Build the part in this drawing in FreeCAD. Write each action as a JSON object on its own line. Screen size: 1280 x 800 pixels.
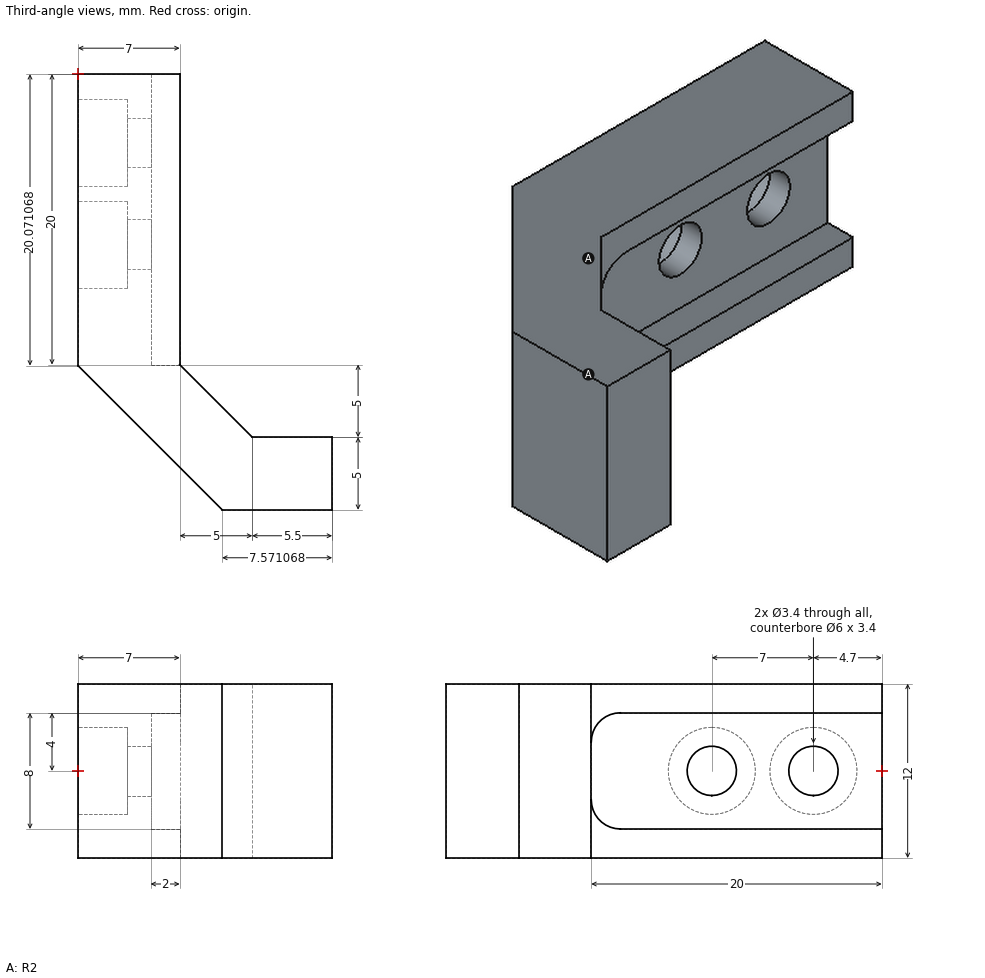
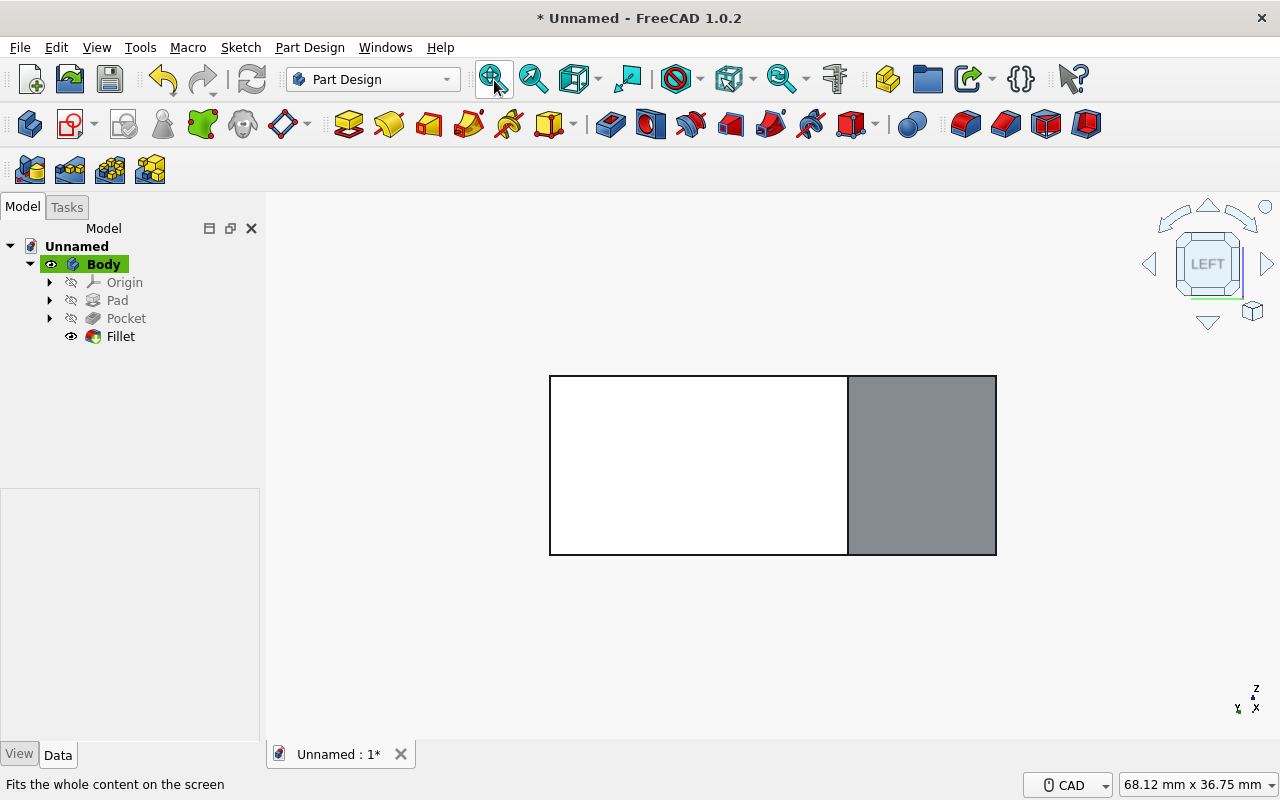
{"action": "left_click", "coordinate": [656, 464]}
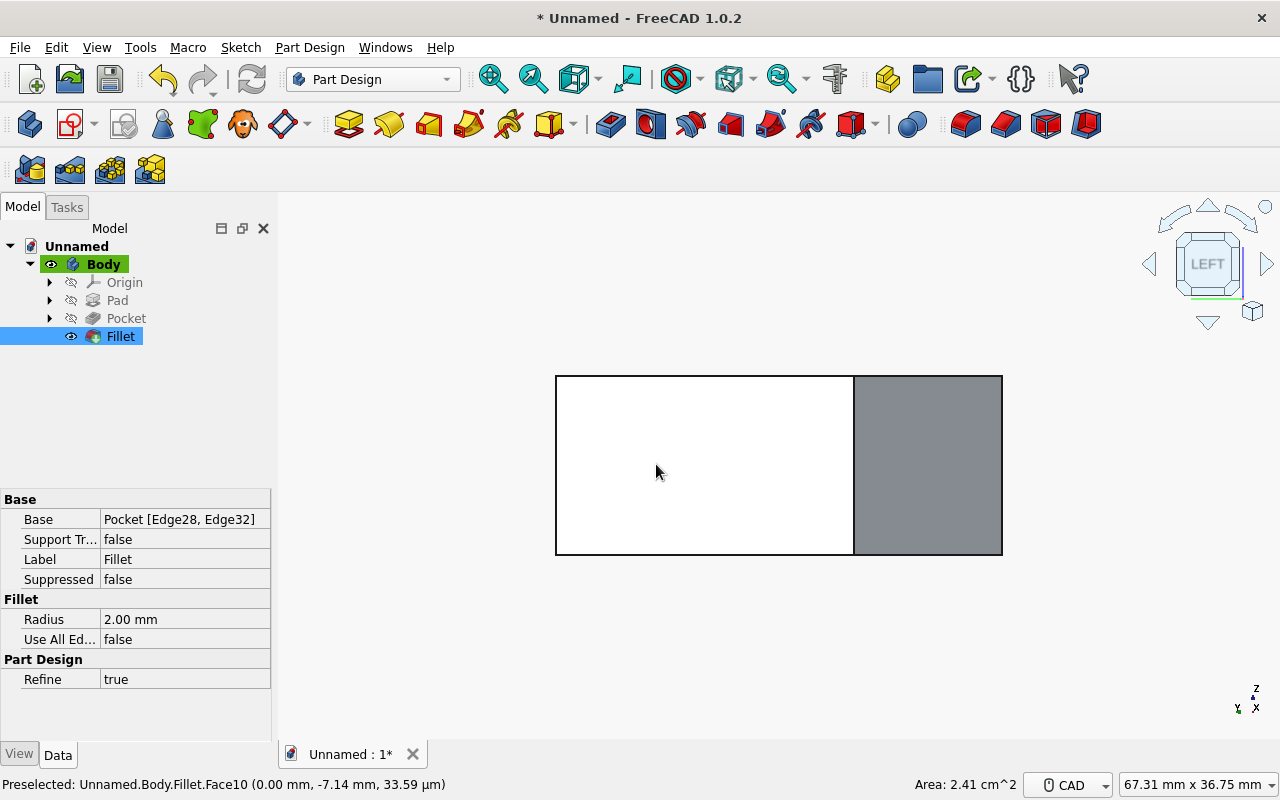
{"action": "left_click", "coordinate": [70, 124]}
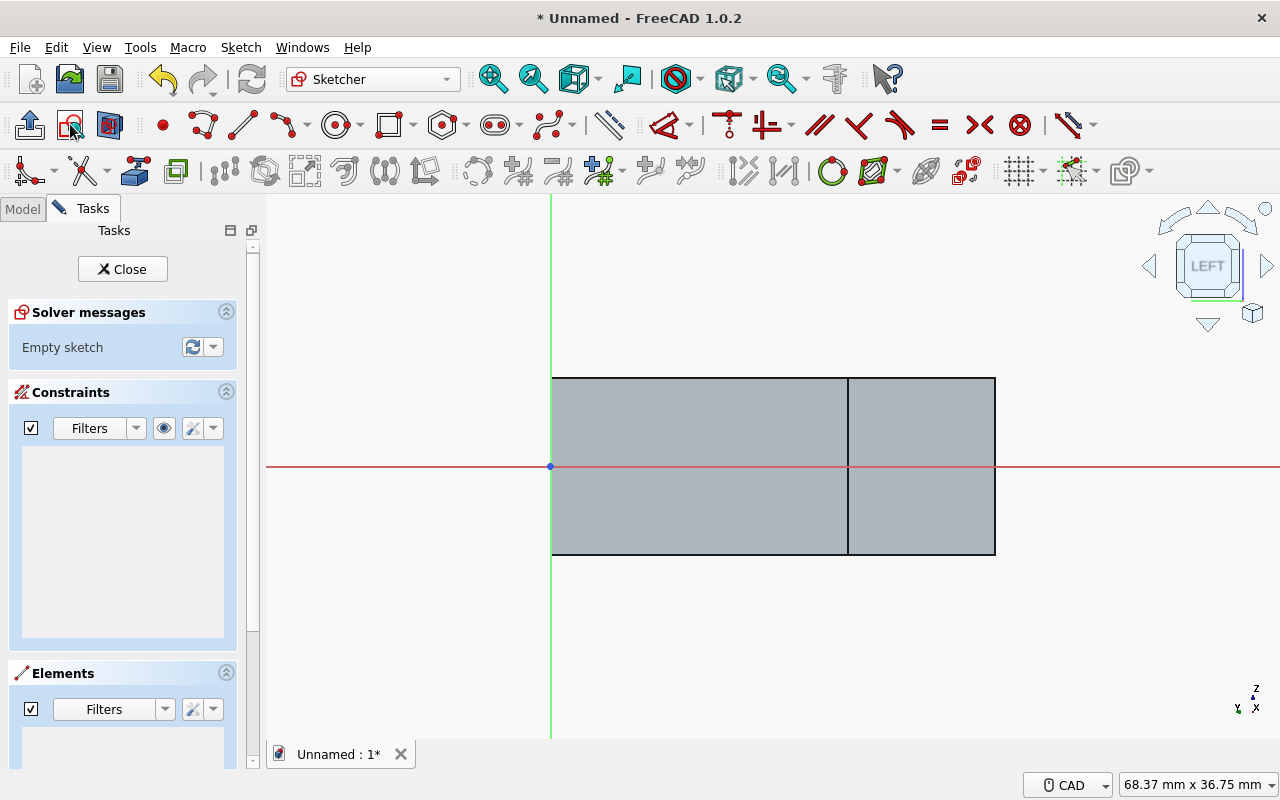
{"action": "scroll", "coordinate": [618, 466], "scroll_direction": "up", "scroll_amount": 5}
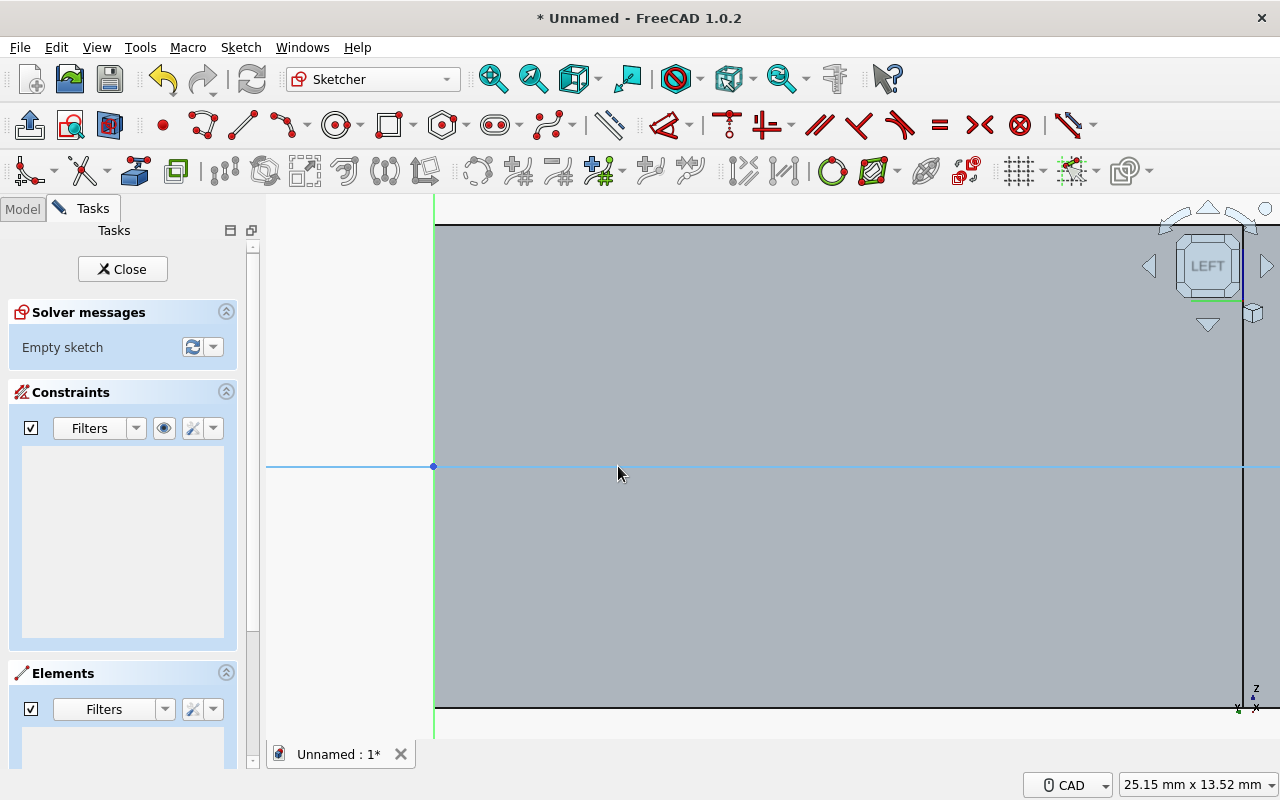
{"action": "left_click", "coordinate": [336, 126]}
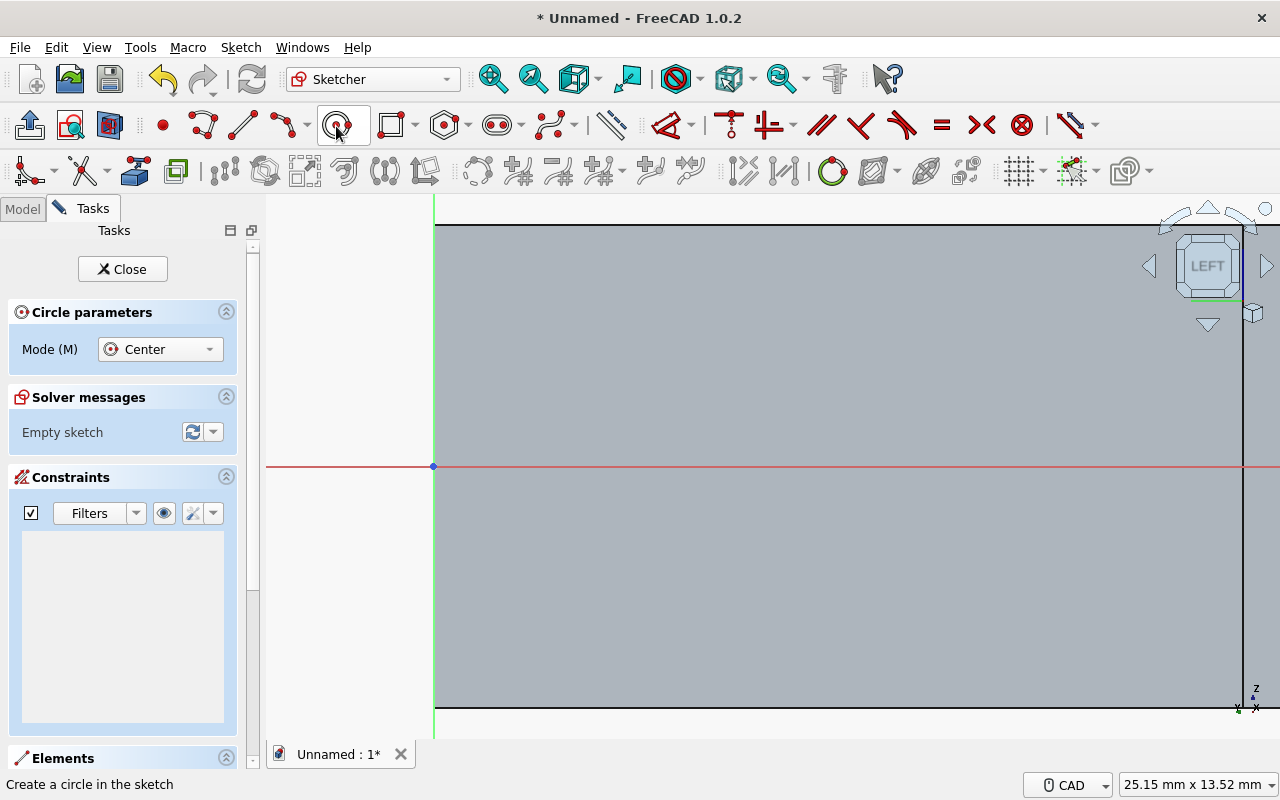
{"action": "left_click", "coordinate": [623, 466]}
{"action": "left_click", "coordinate": [672, 418]}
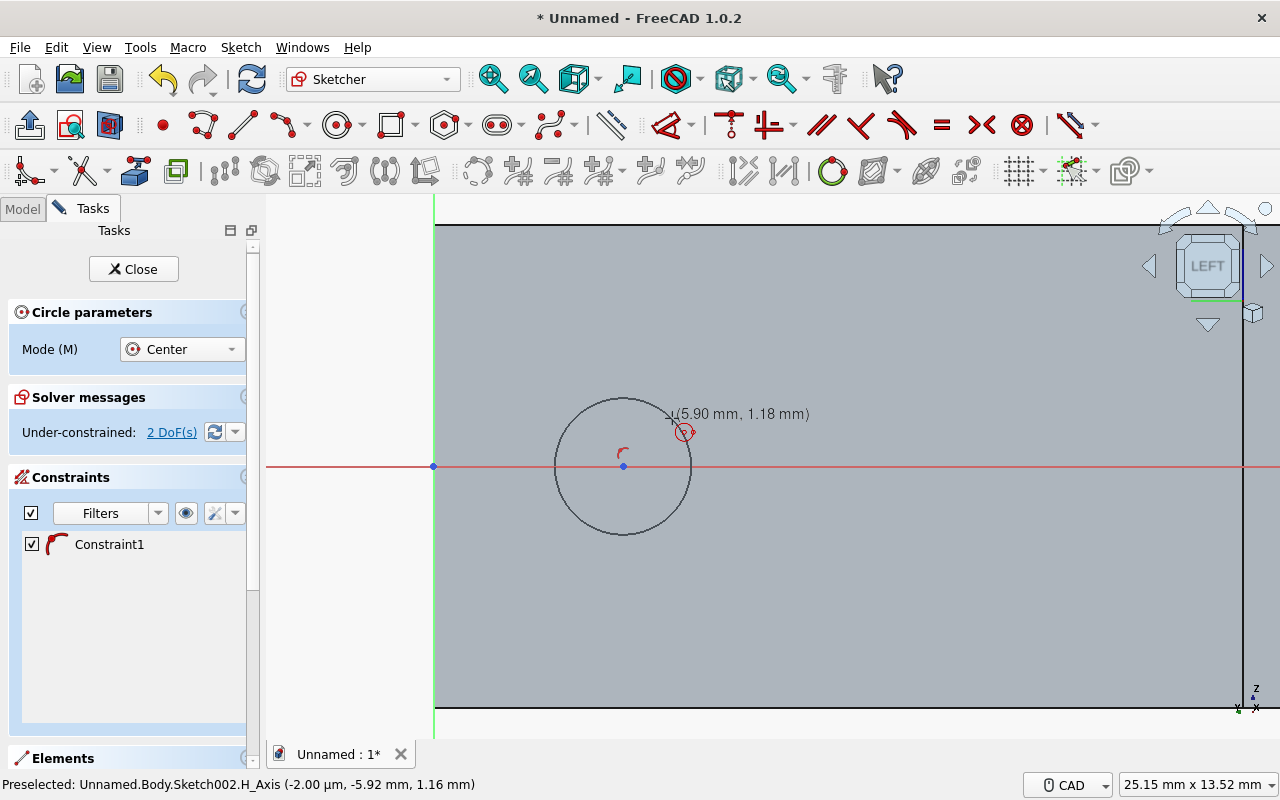
{"action": "left_click", "coordinate": [906, 466]}
{"action": "left_click", "coordinate": [954, 418]}
{"action": "key", "text": "Escape"}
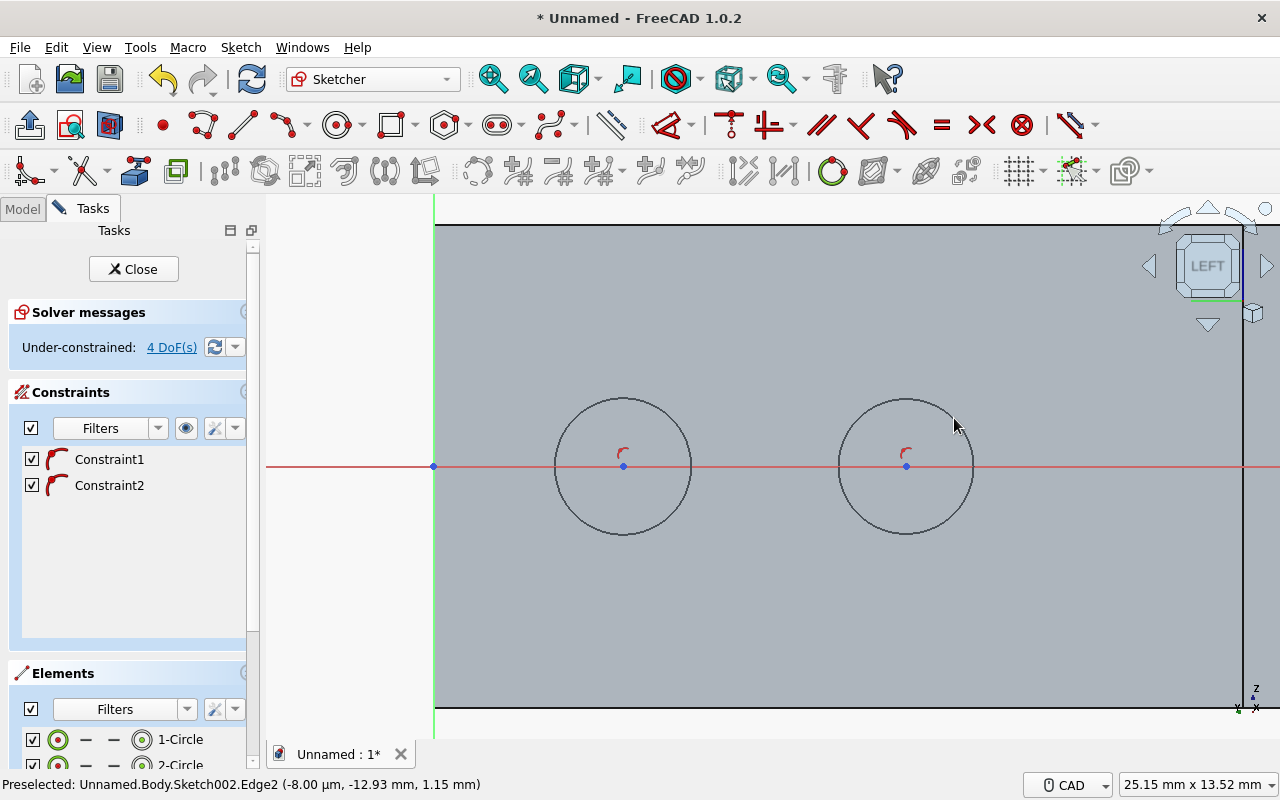
{"action": "left_click", "coordinate": [671, 418]}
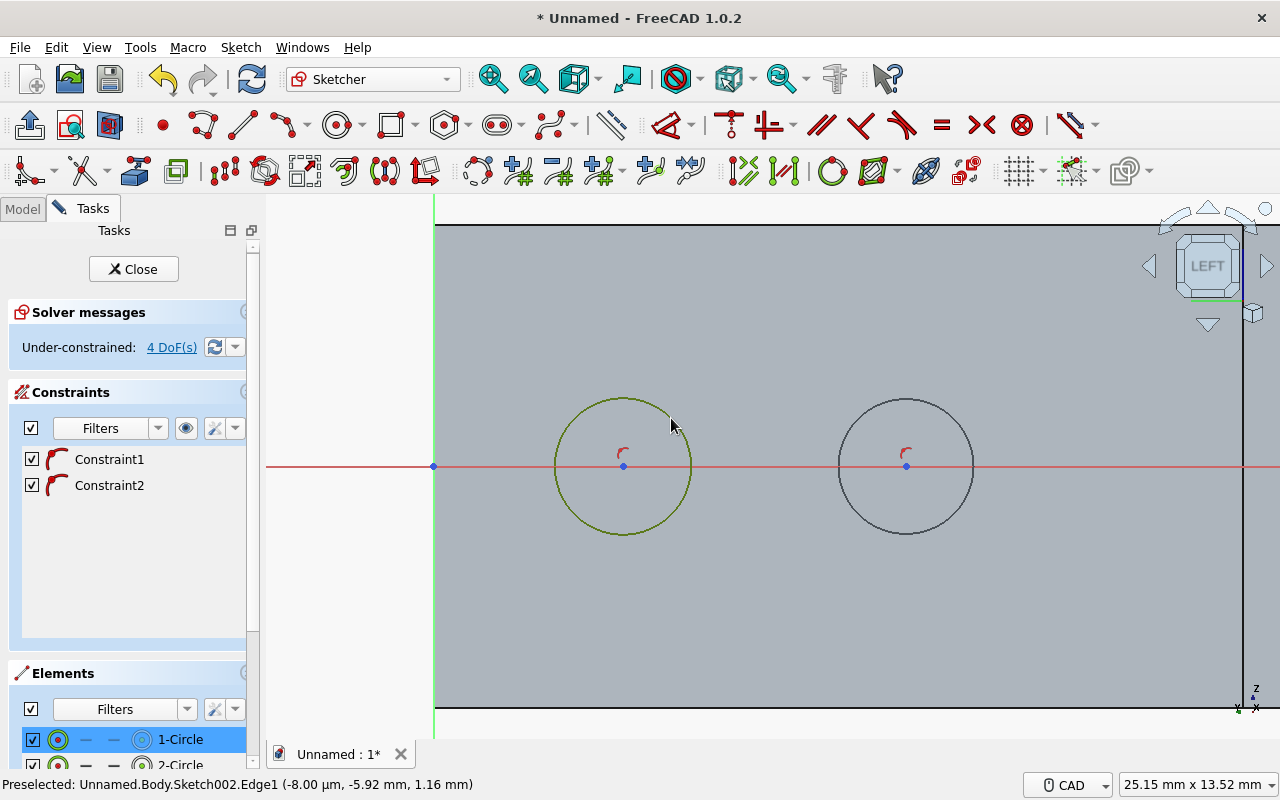
{"action": "left_click", "coordinate": [954, 419]}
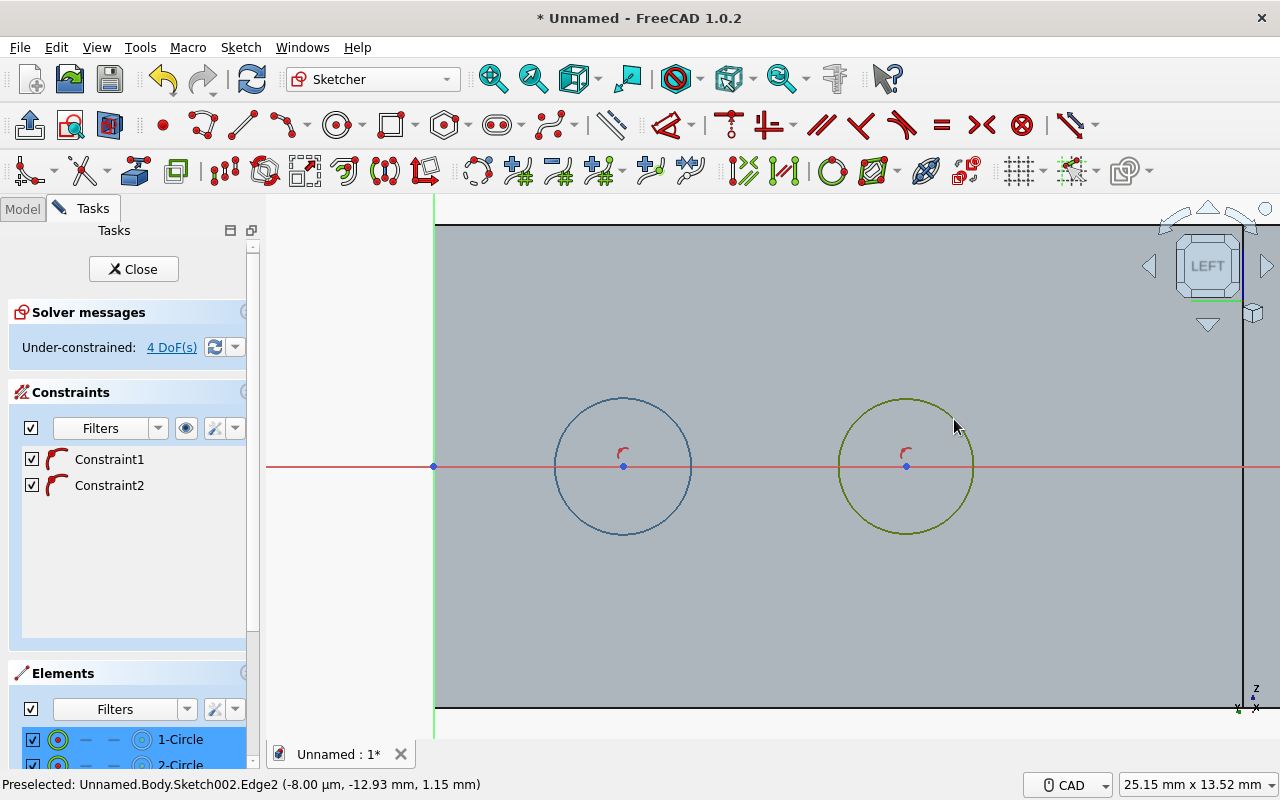
{"action": "left_click", "coordinate": [942, 126]}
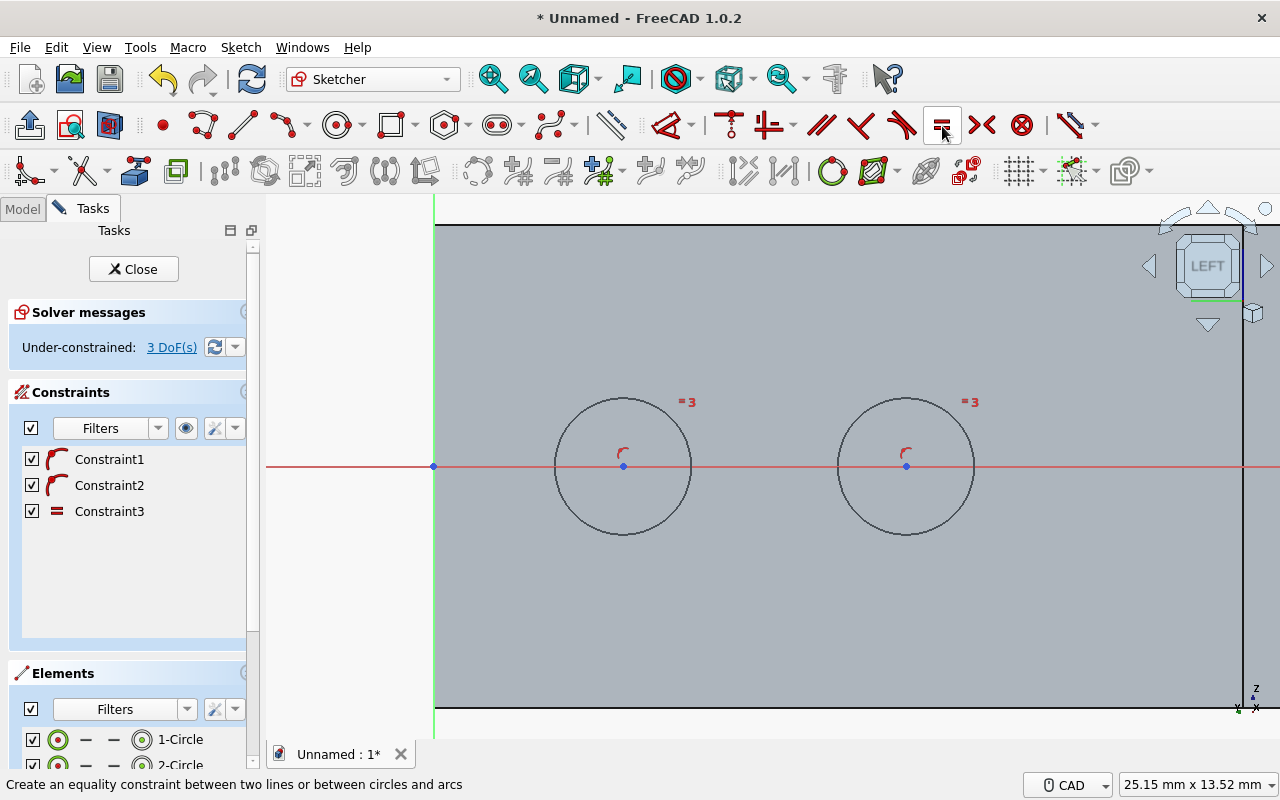
{"action": "left_click", "coordinate": [666, 126]}